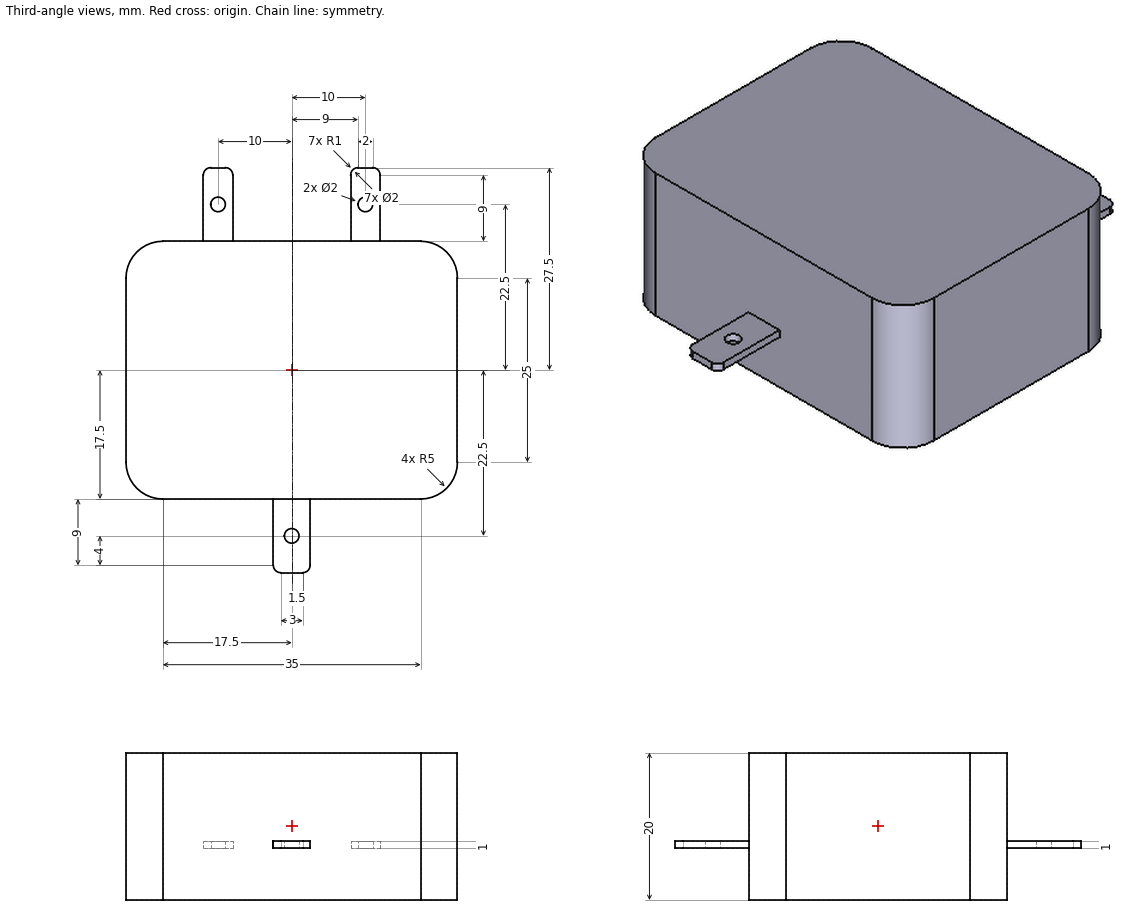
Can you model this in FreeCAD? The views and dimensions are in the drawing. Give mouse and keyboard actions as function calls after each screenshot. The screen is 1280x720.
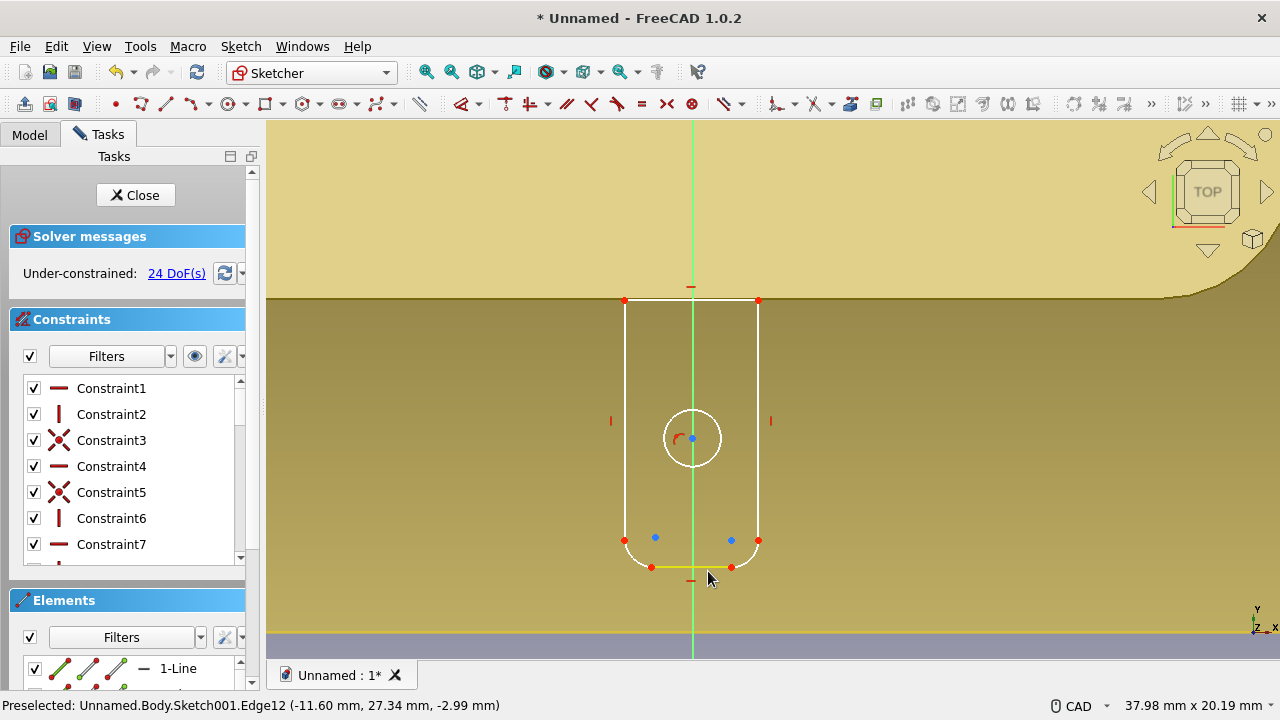
click(708, 567)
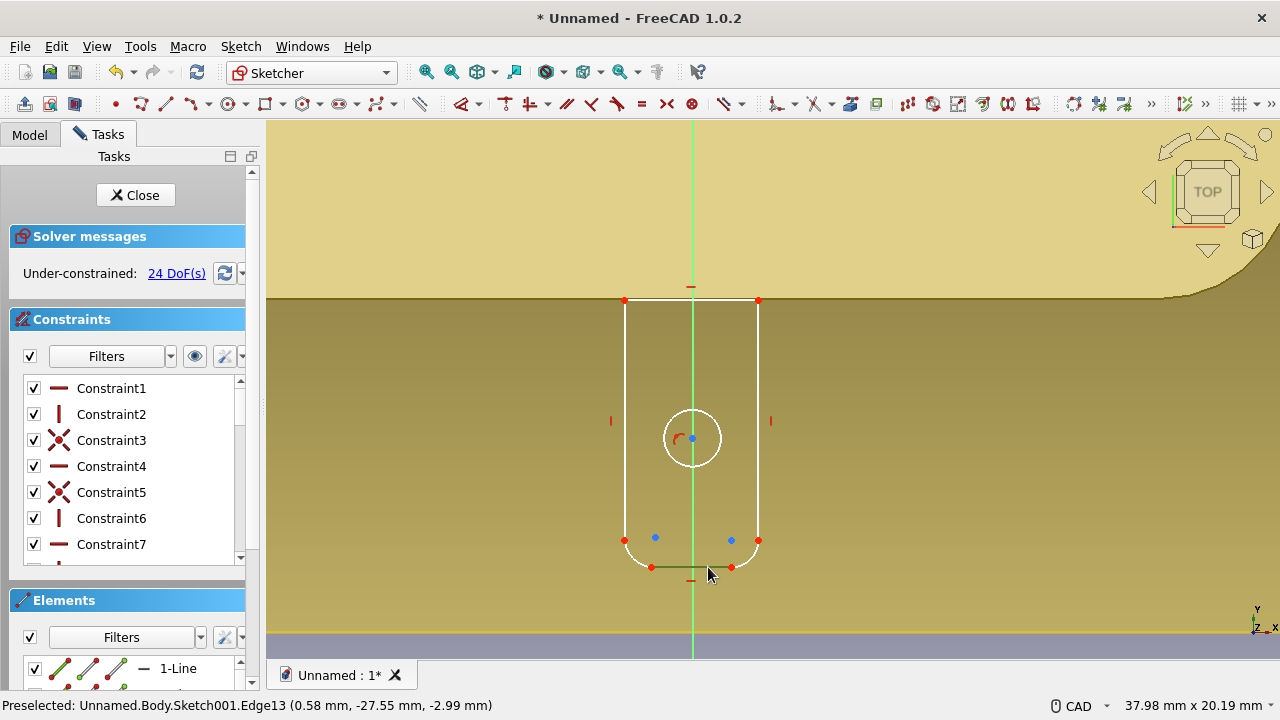
click(629, 552)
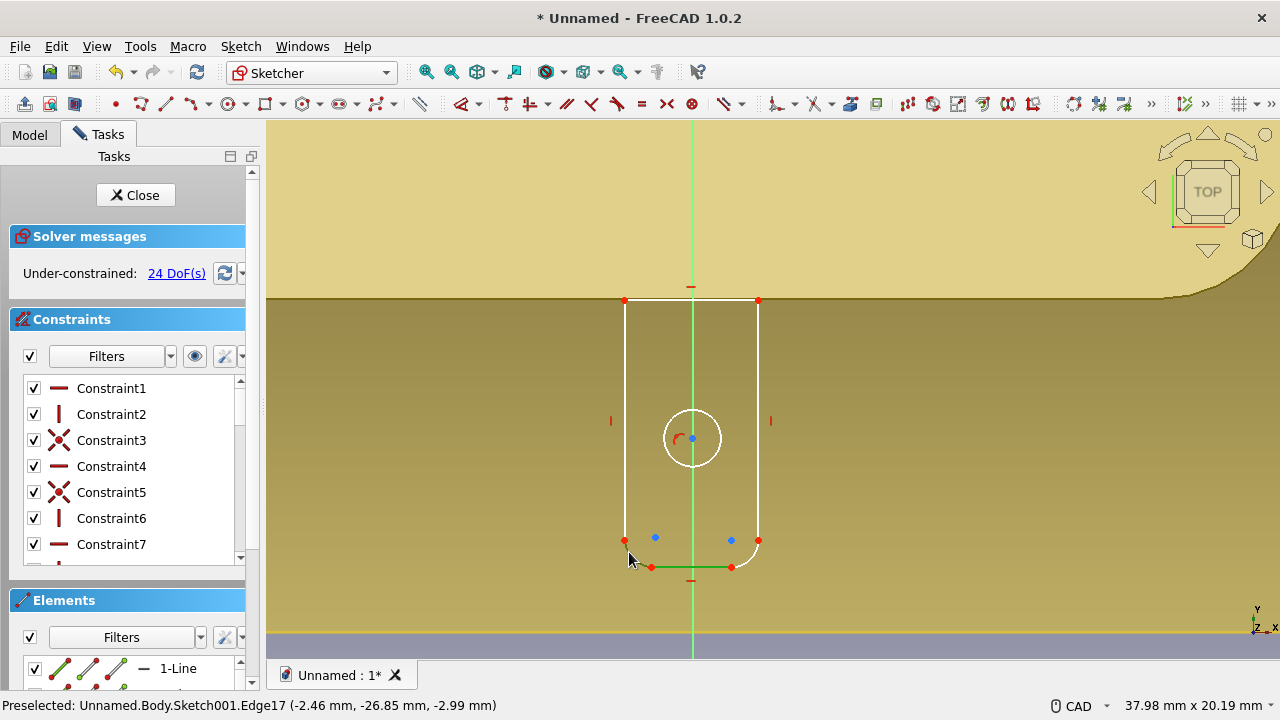
key(t)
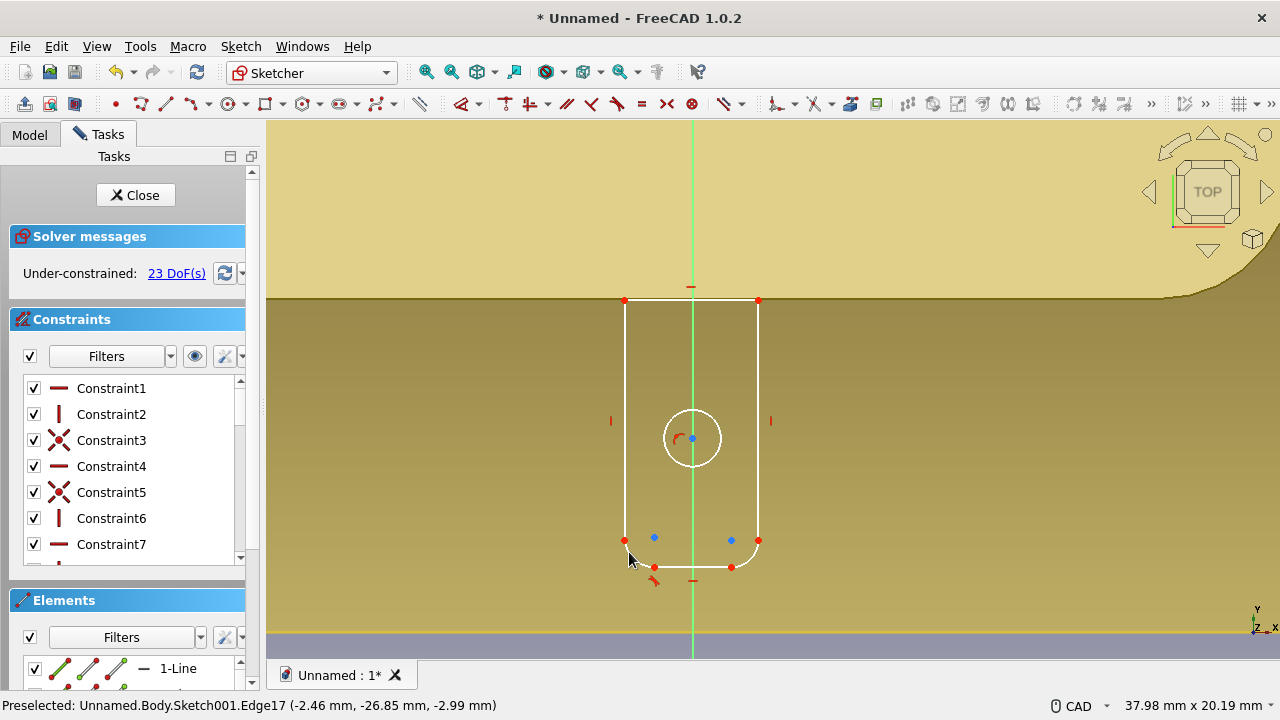
click(709, 567)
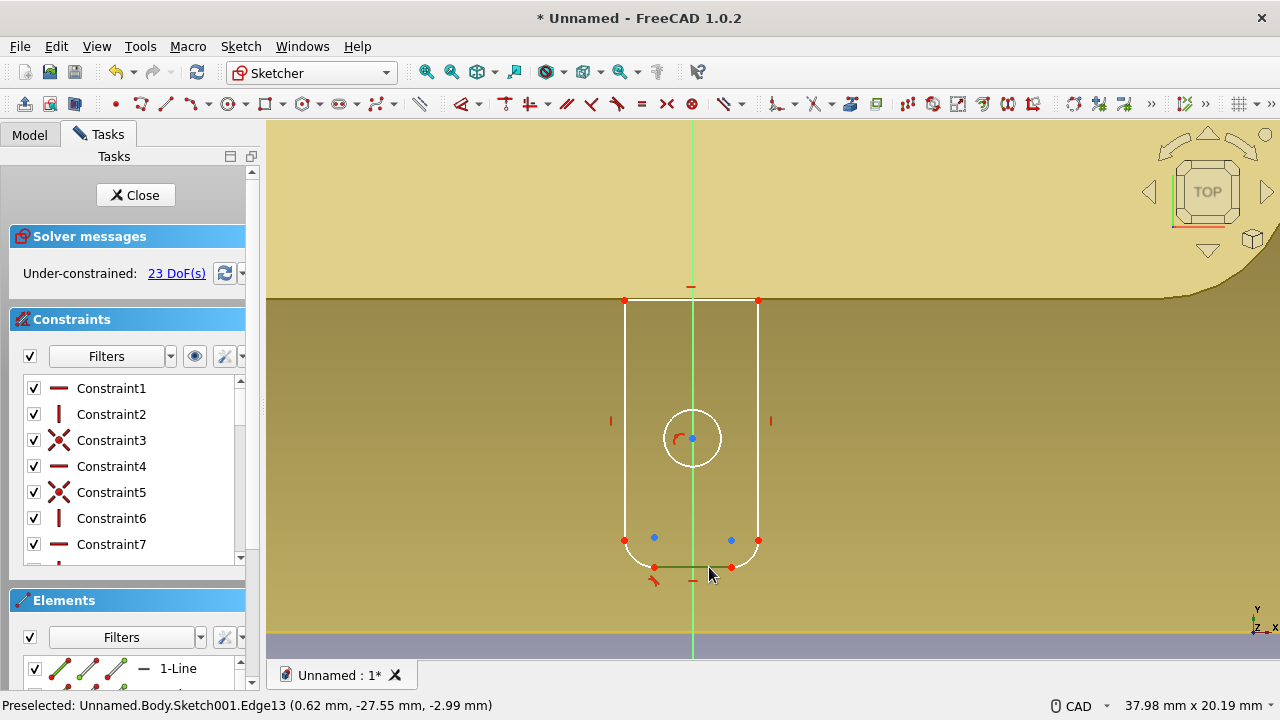
click(744, 564)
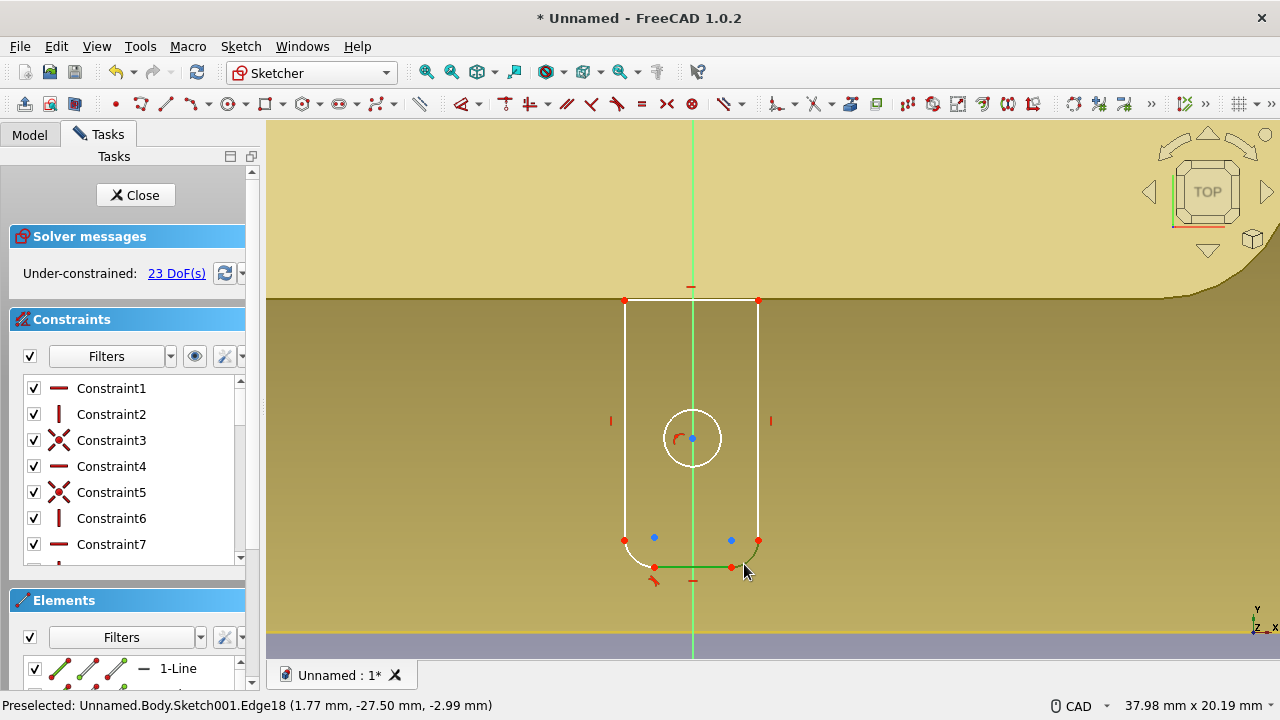
click(617, 104)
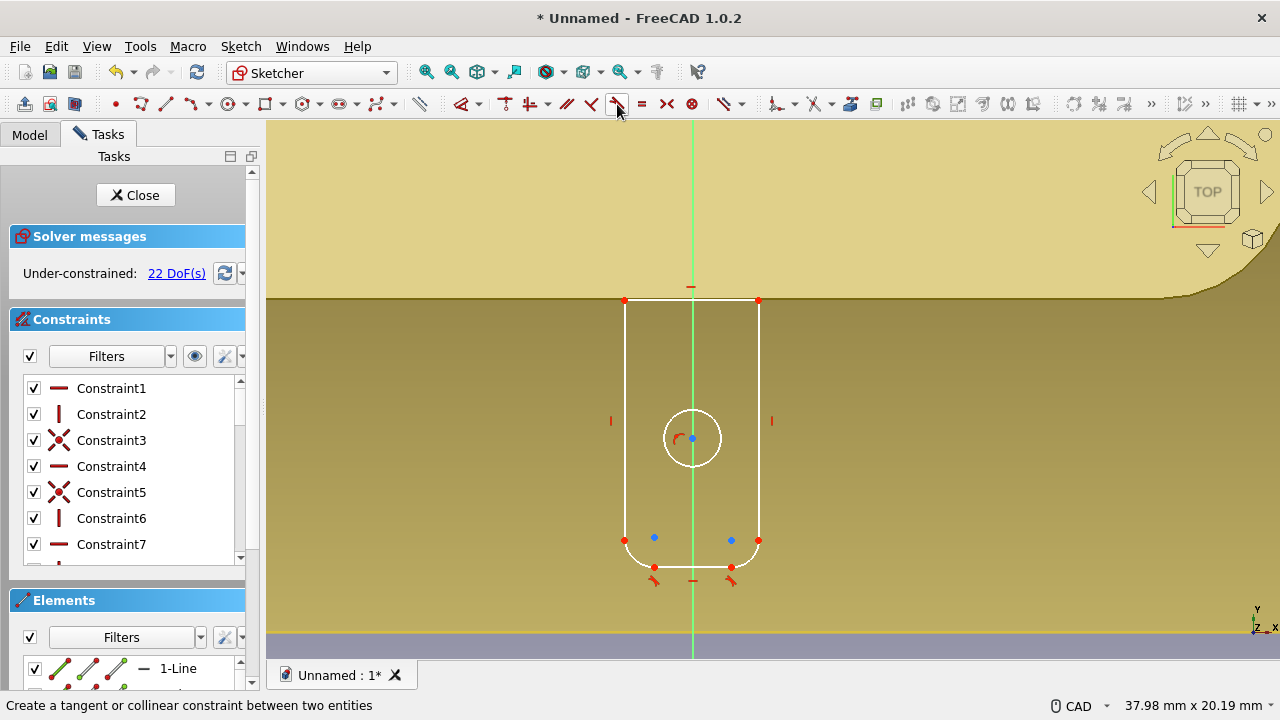
scroll(708, 572, down, 7)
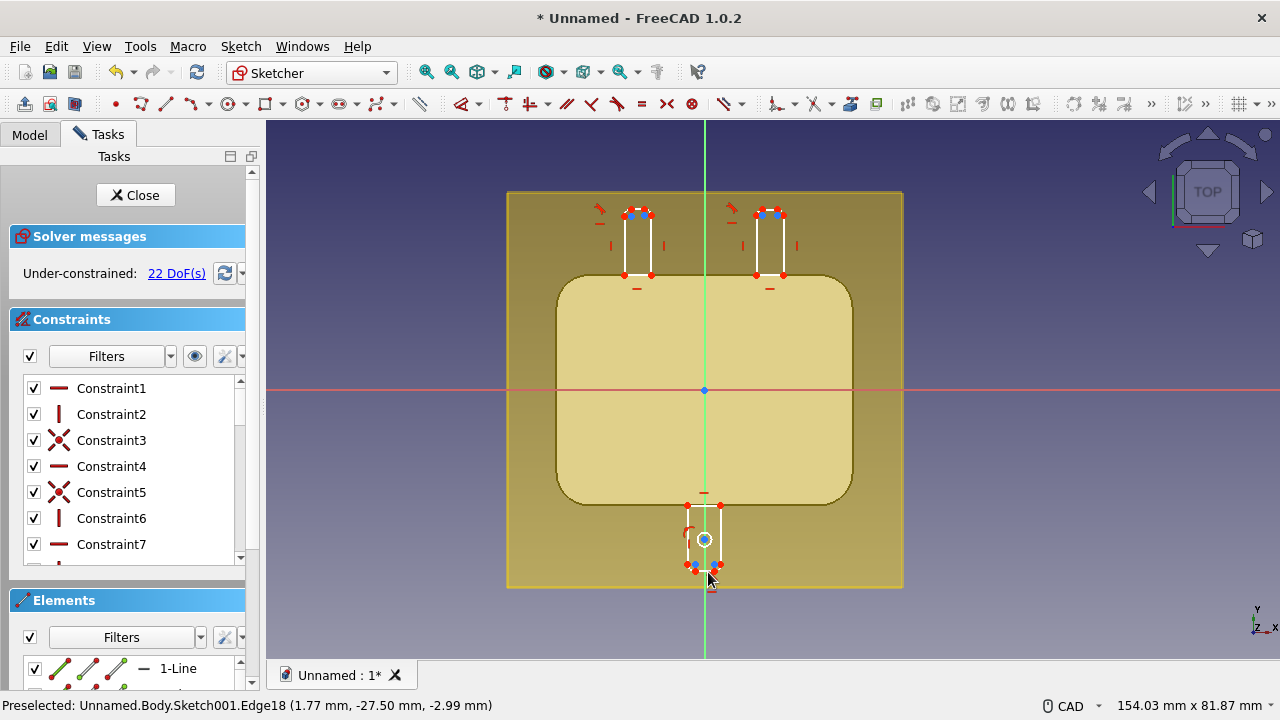
scroll(688, 547, up, 2)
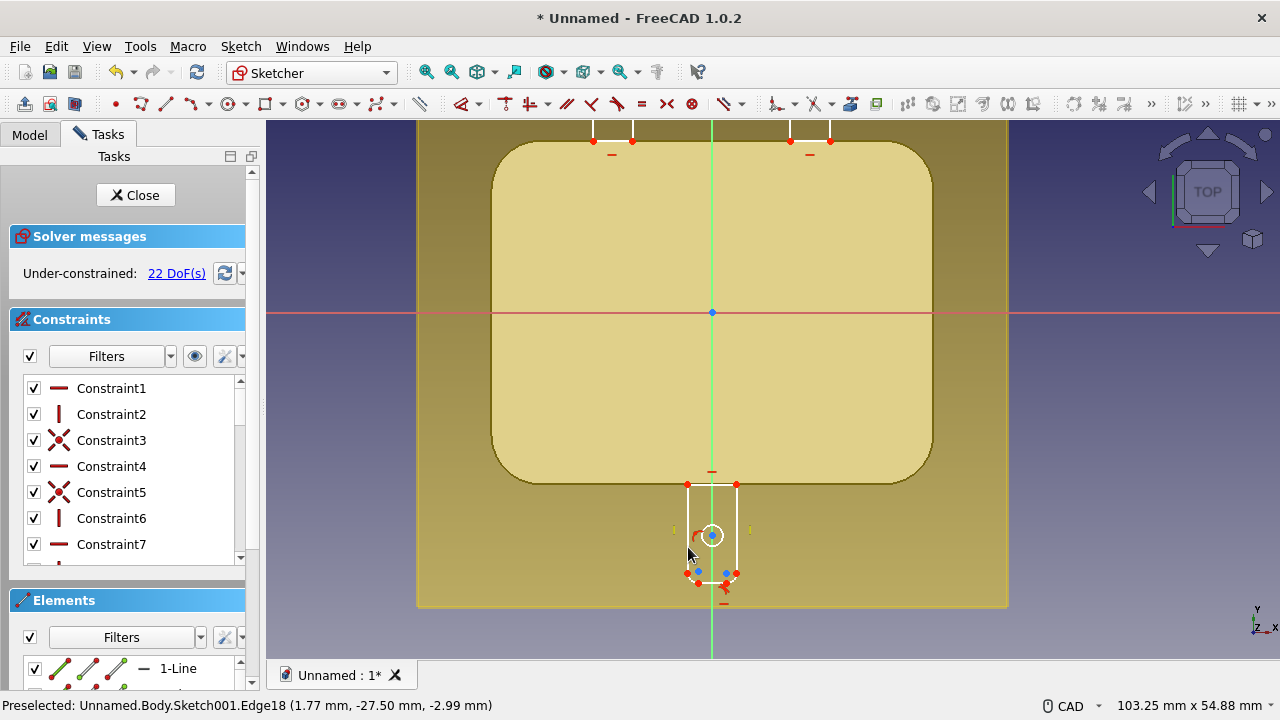
click(688, 547)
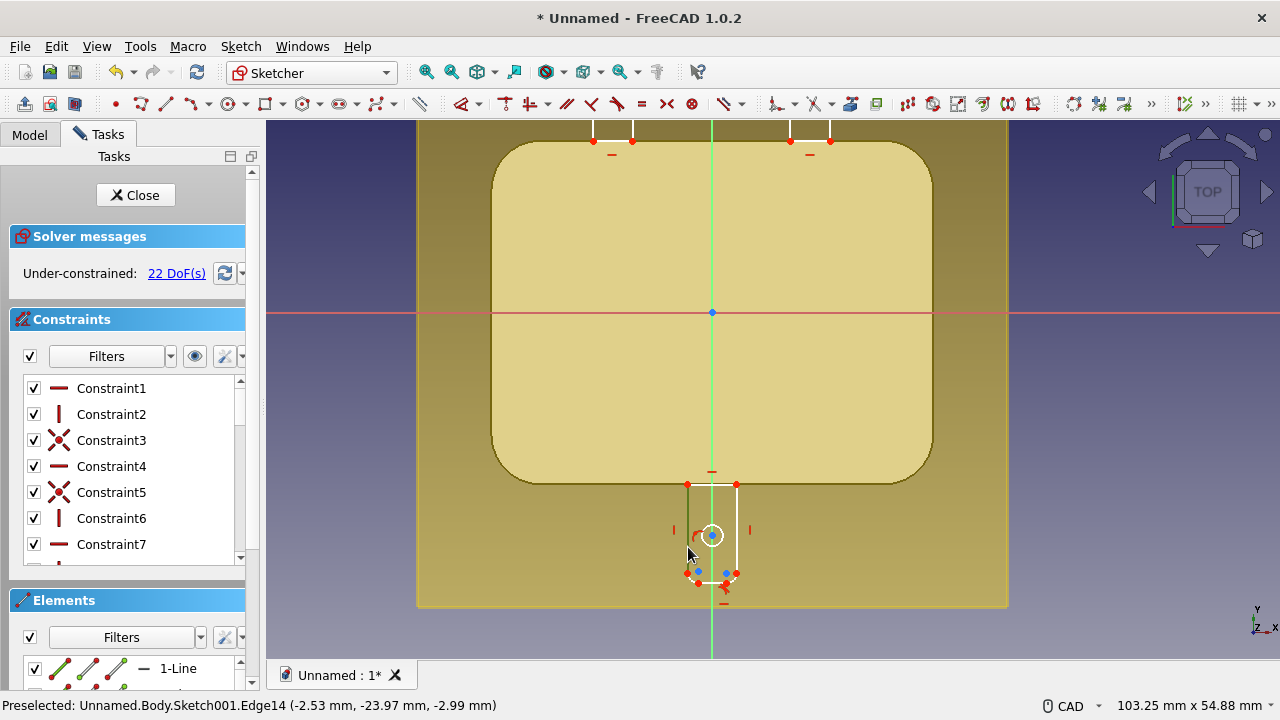
scroll(691, 580, up, 3)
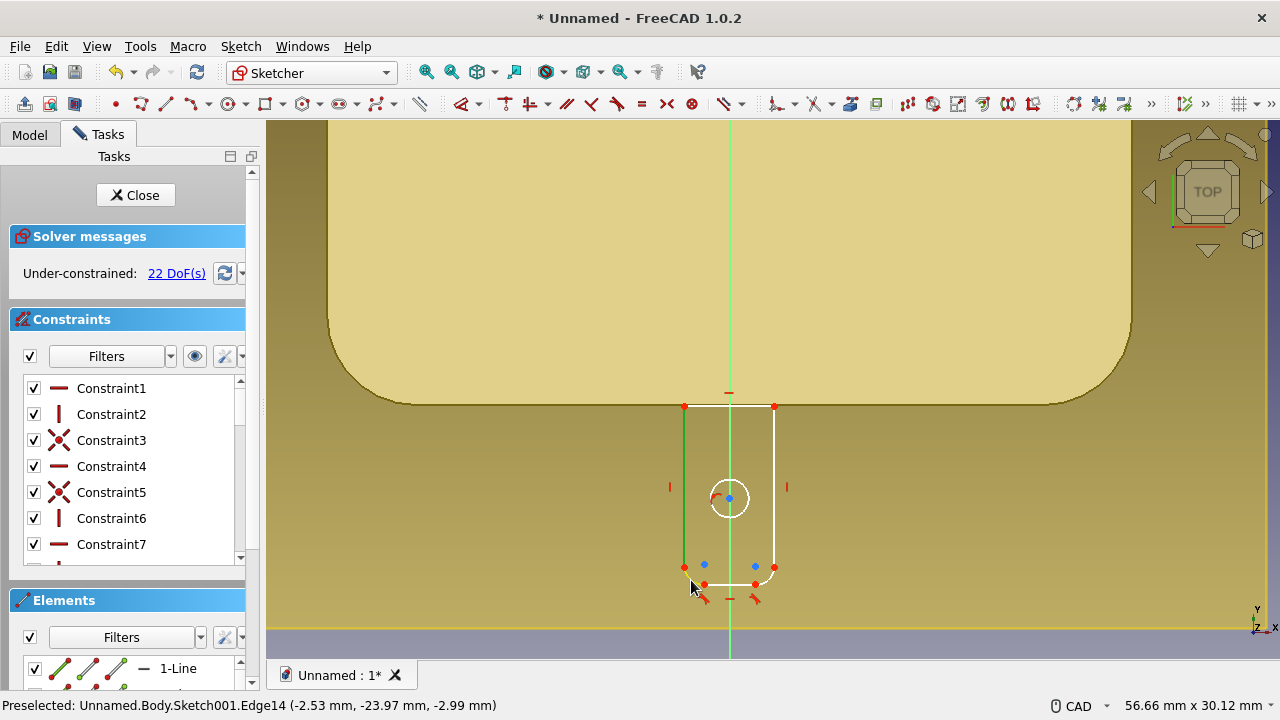
click(691, 580)